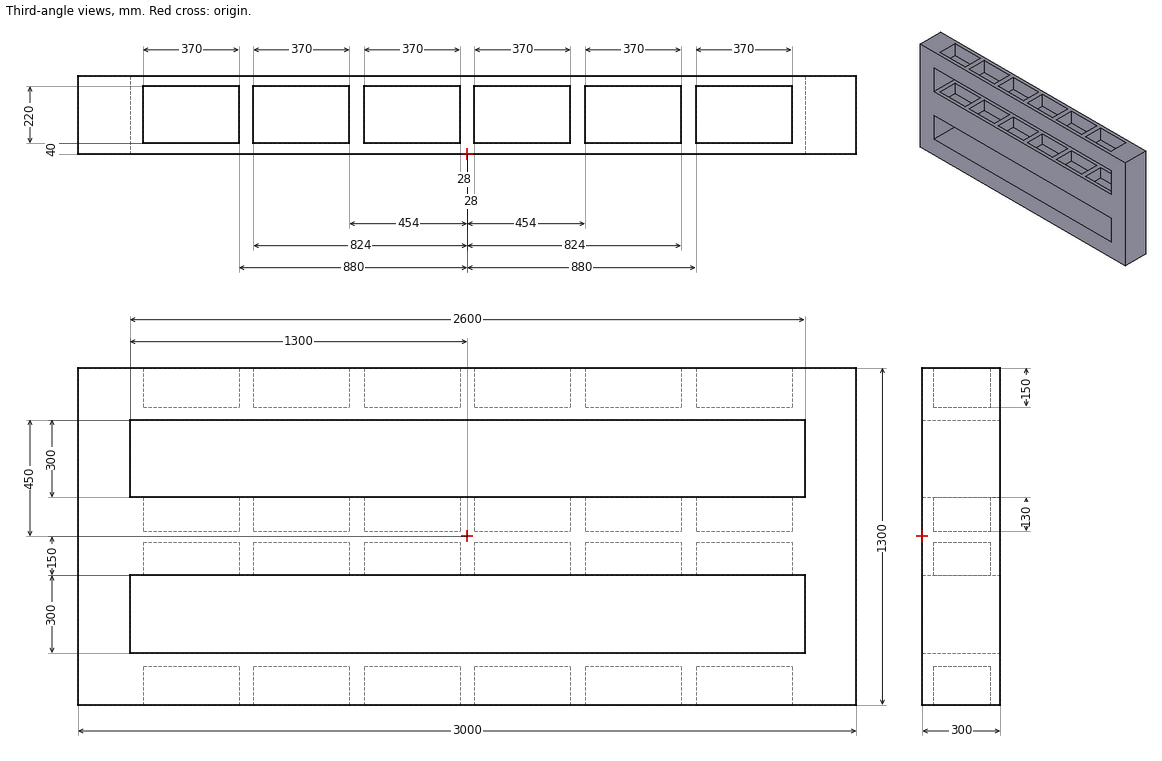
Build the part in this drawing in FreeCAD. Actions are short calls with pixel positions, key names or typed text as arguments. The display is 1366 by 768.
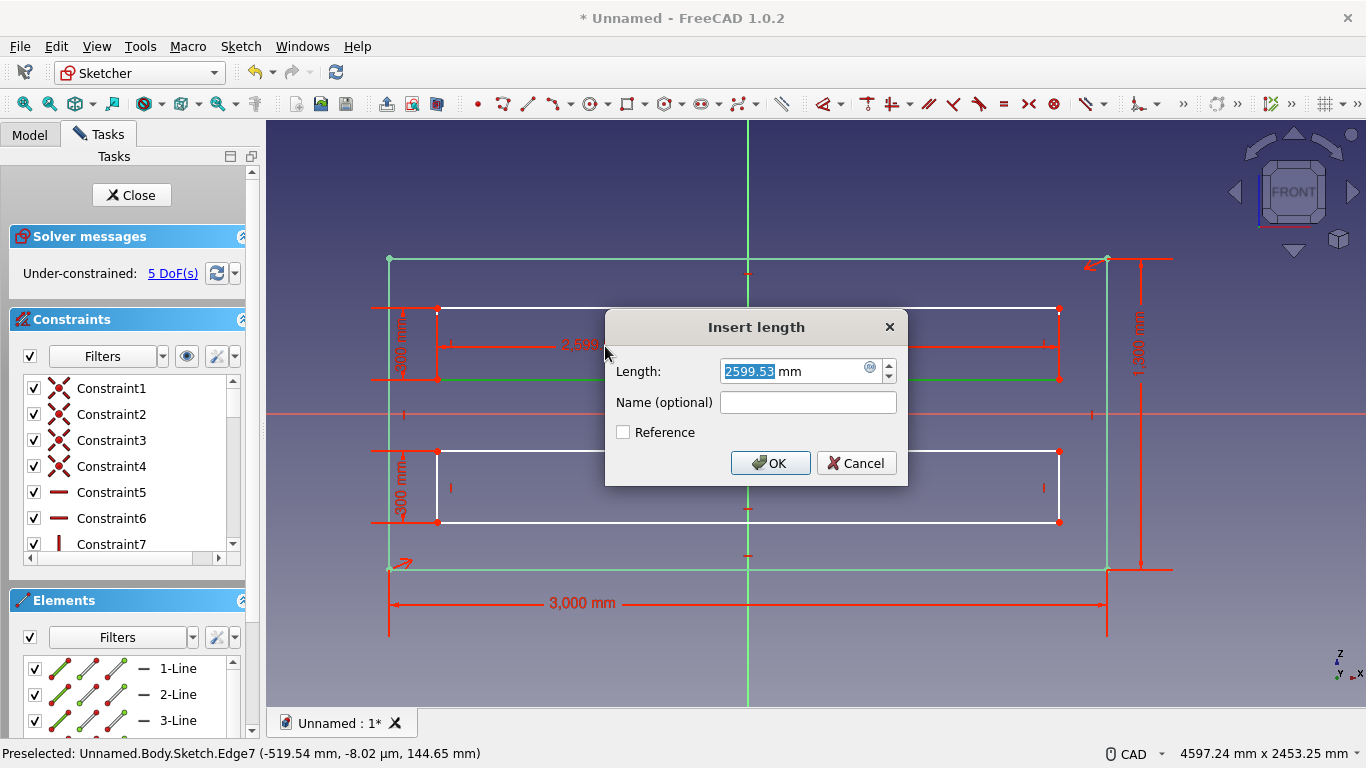
text(2600)
key(Return)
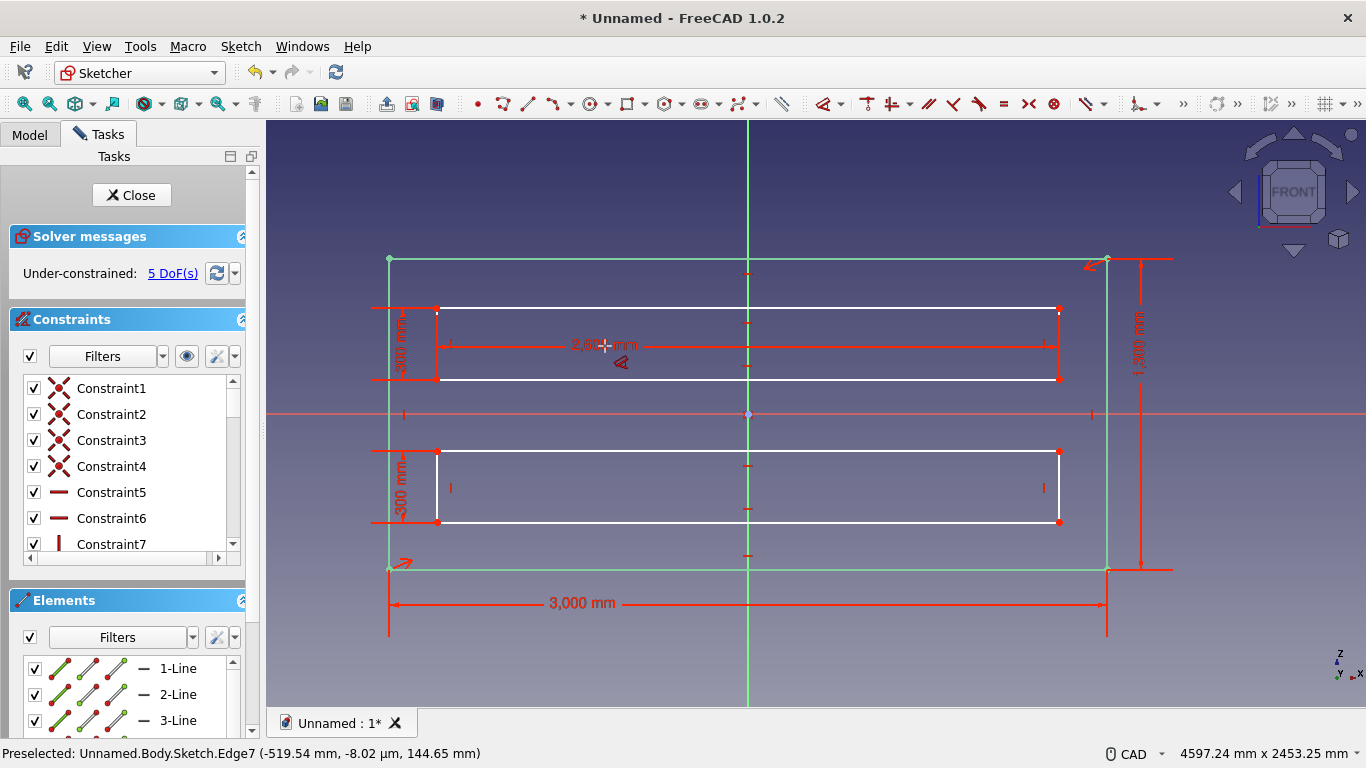
click(624, 523)
click(605, 557)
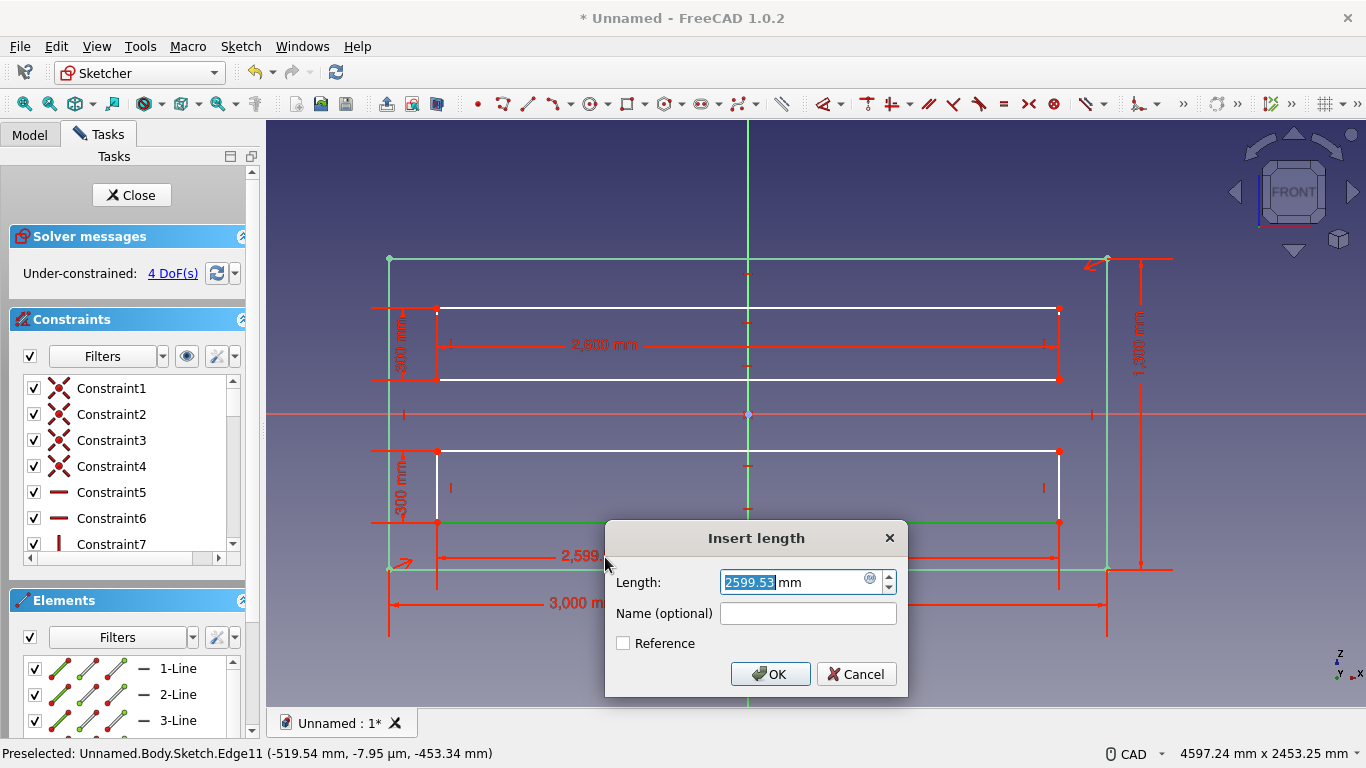
text(2600)
key(Return)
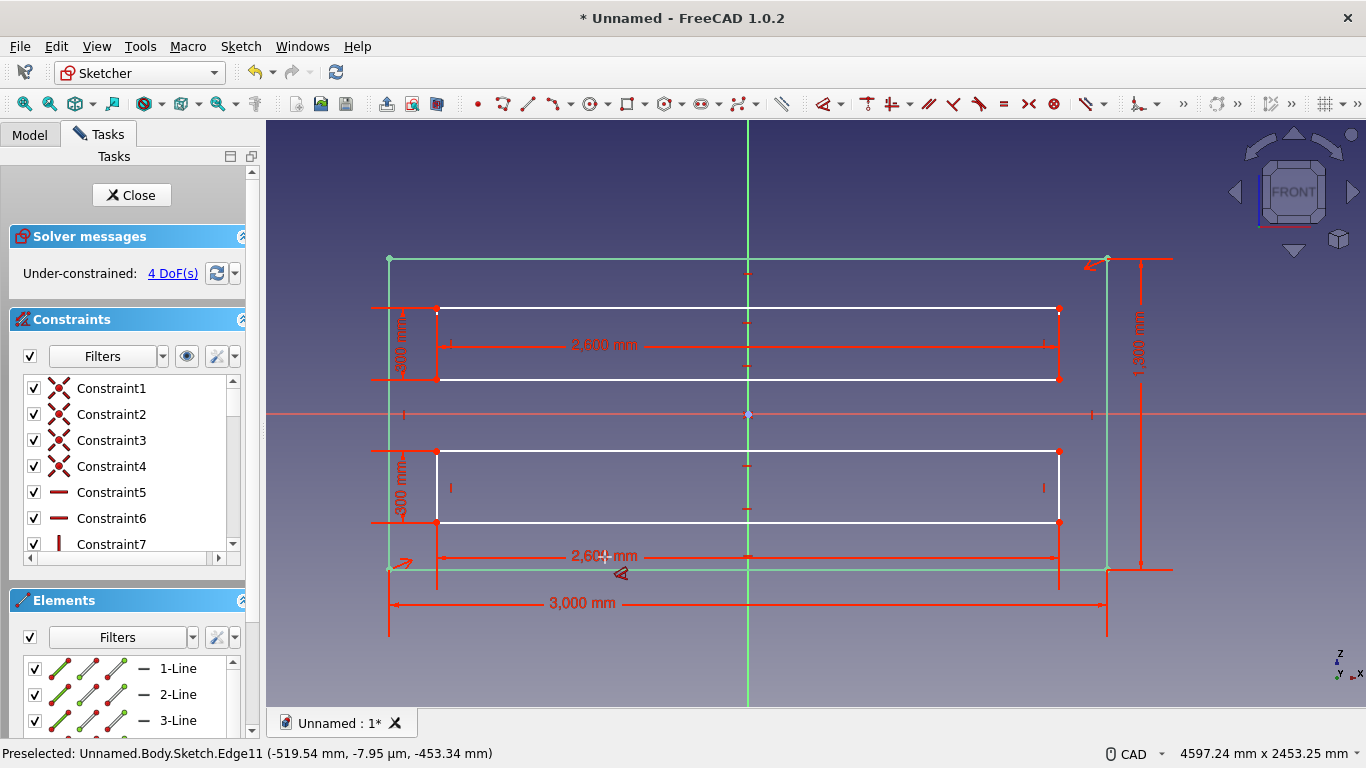
click(437, 308)
click(403, 386)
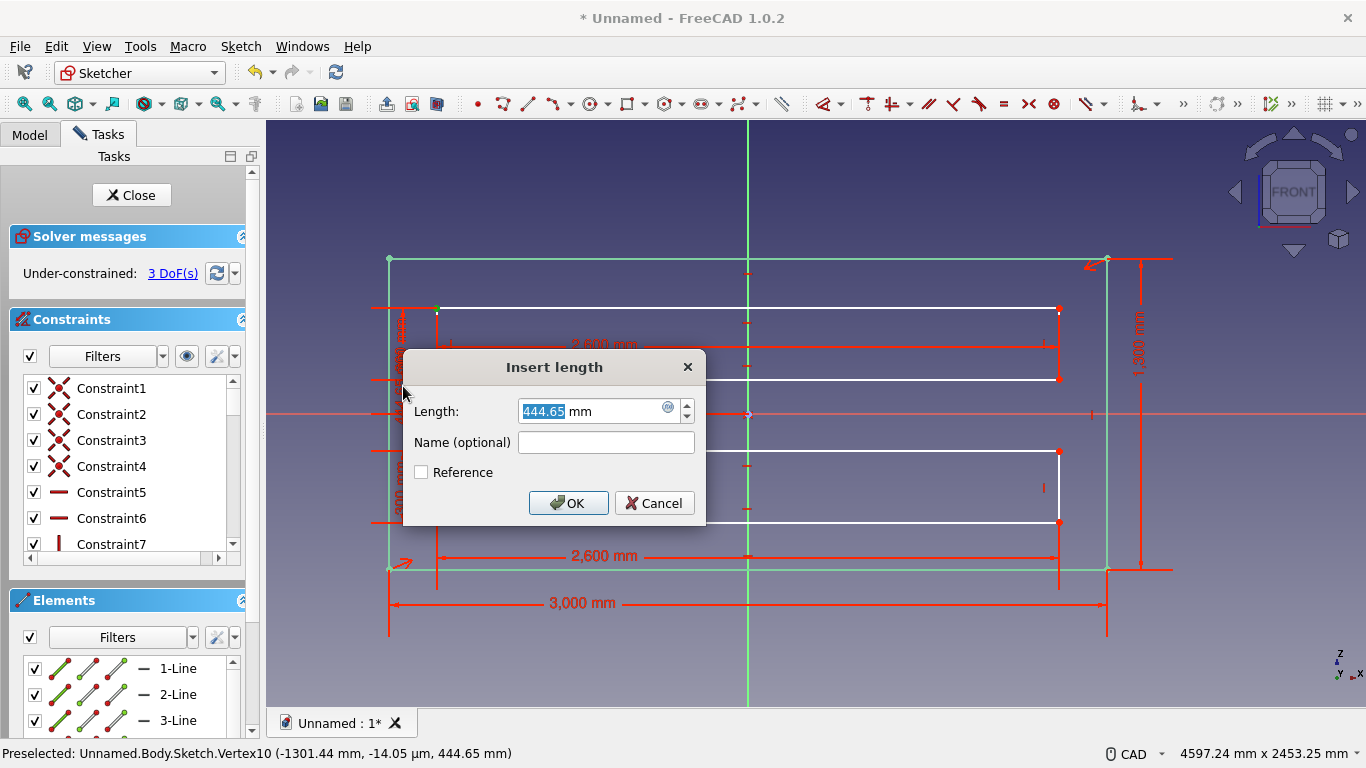
text(450)
key(Return)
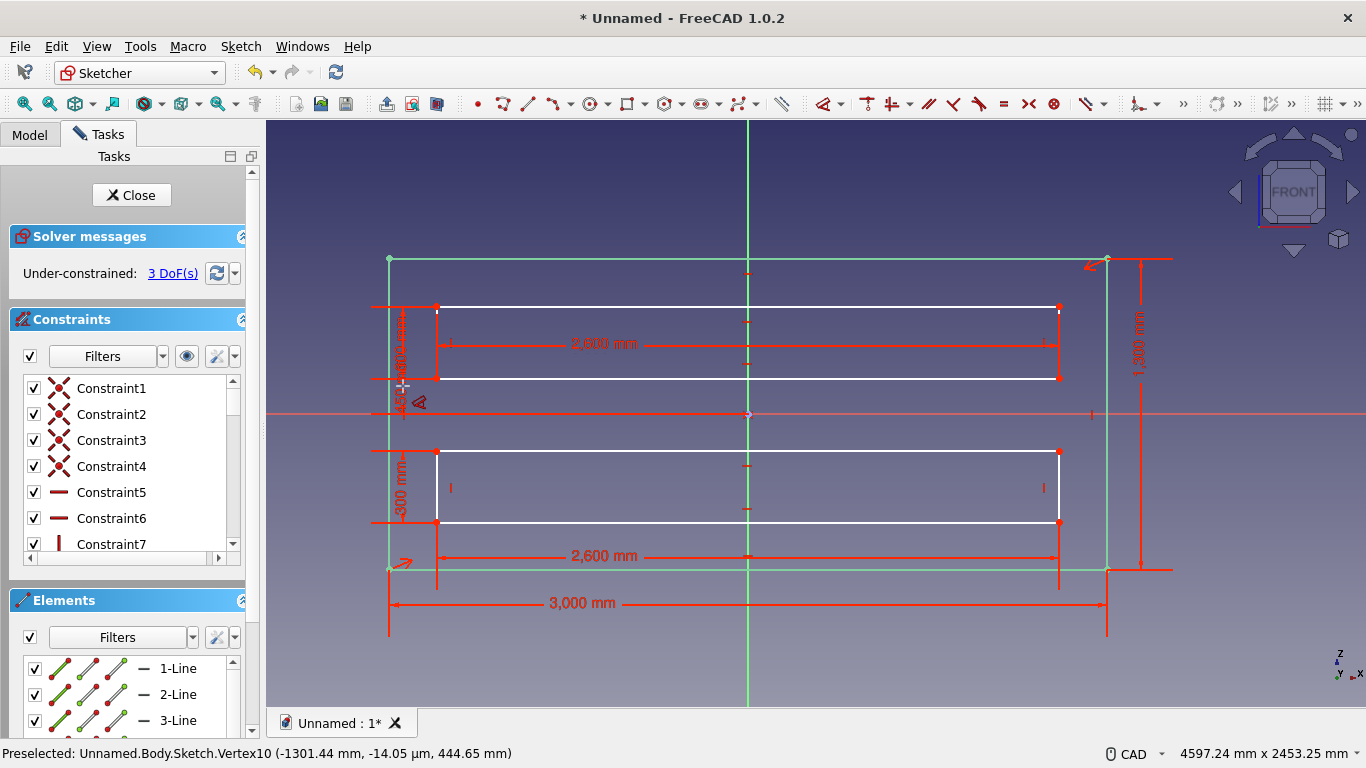
click(437, 451)
click(403, 433)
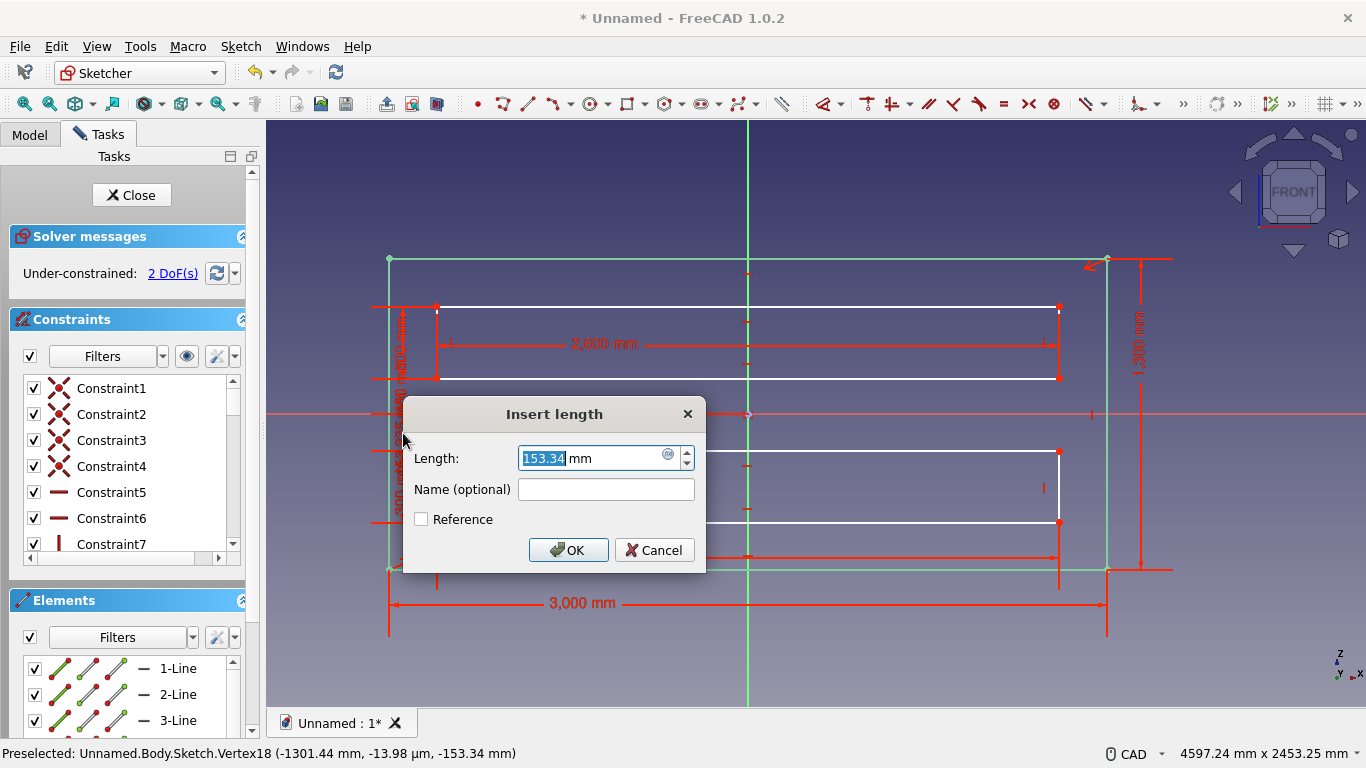
text(150)
key(Return)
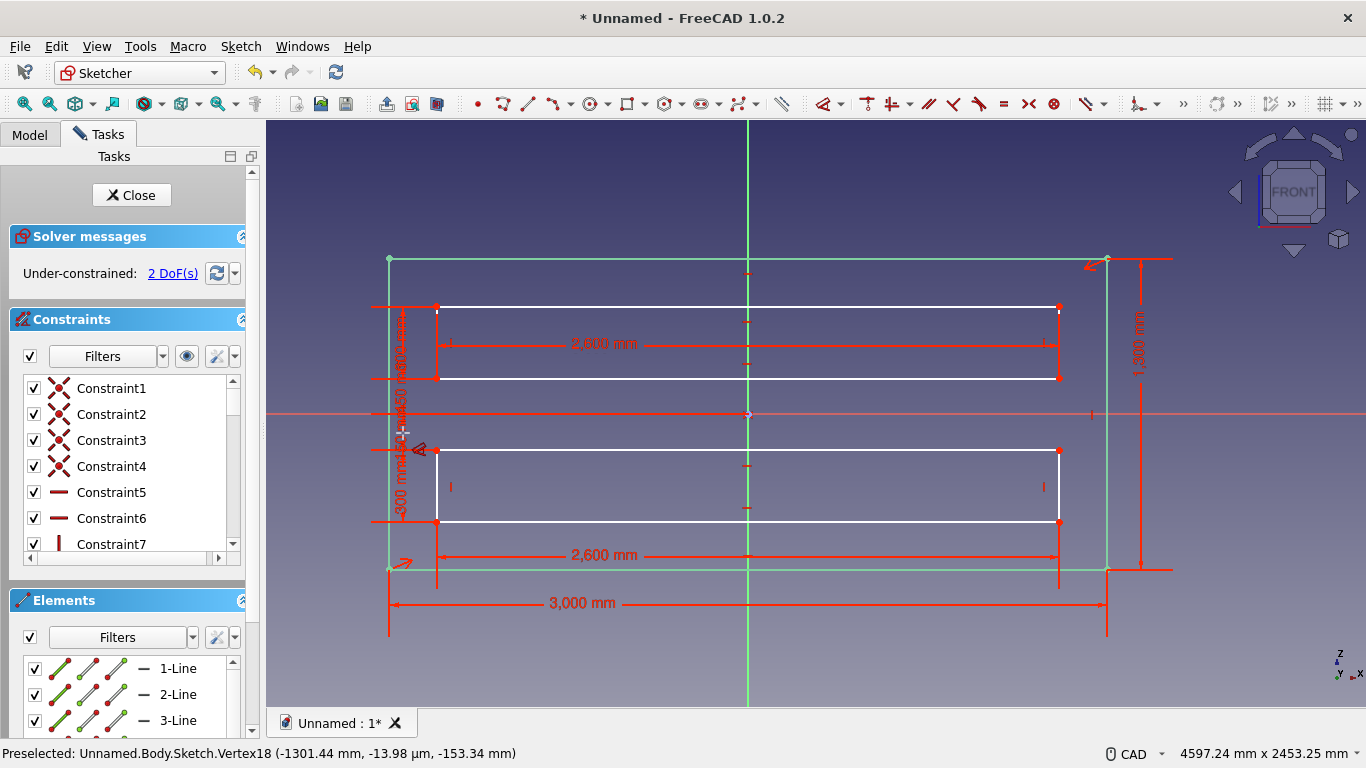
click(437, 307)
click(593, 273)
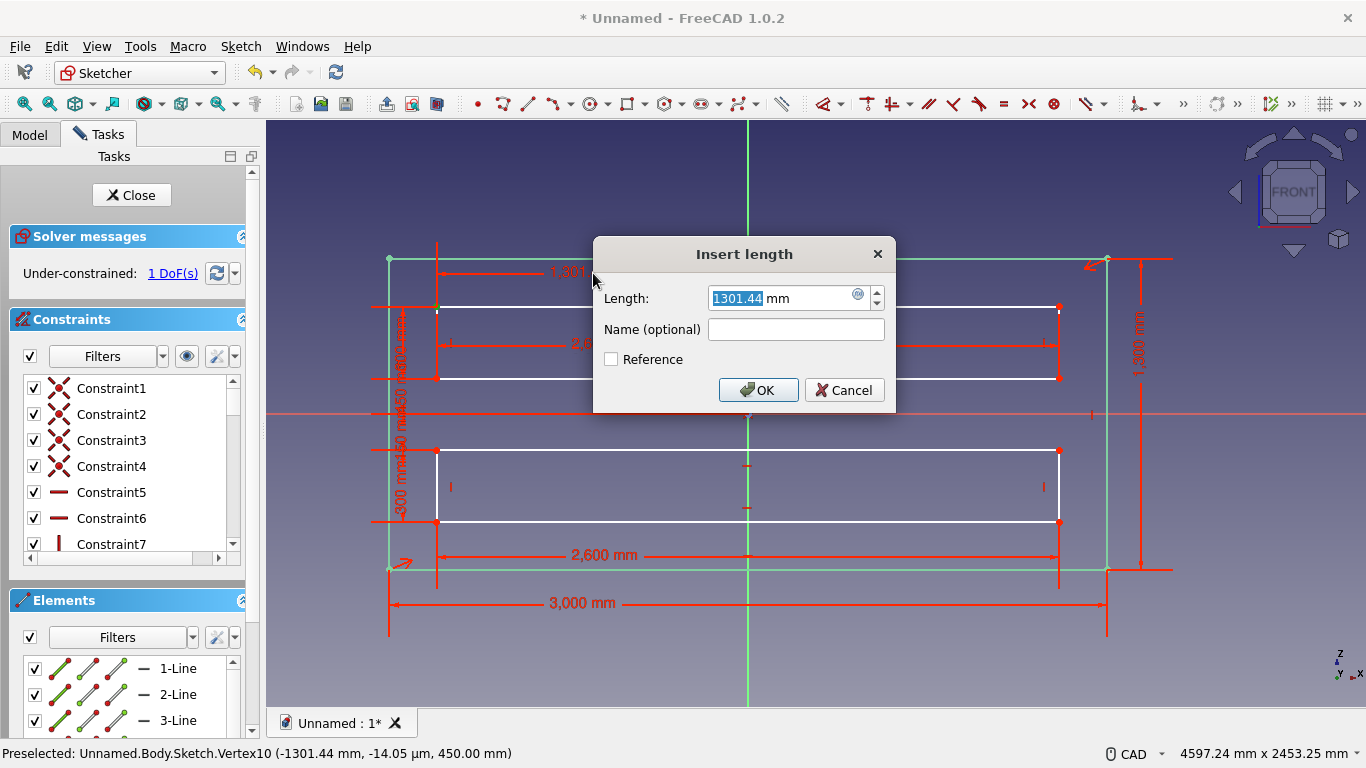
text(1300)
key(Return)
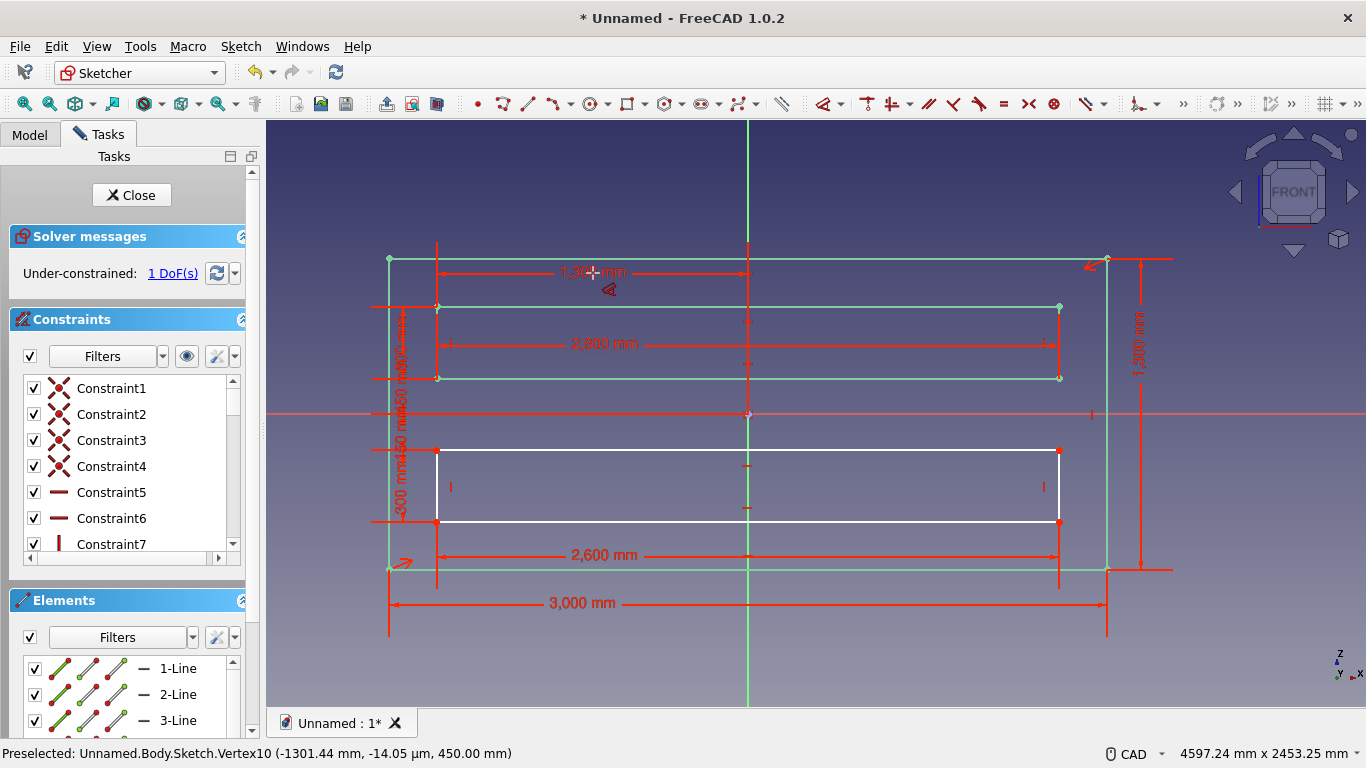
click(437, 450)
click(593, 484)